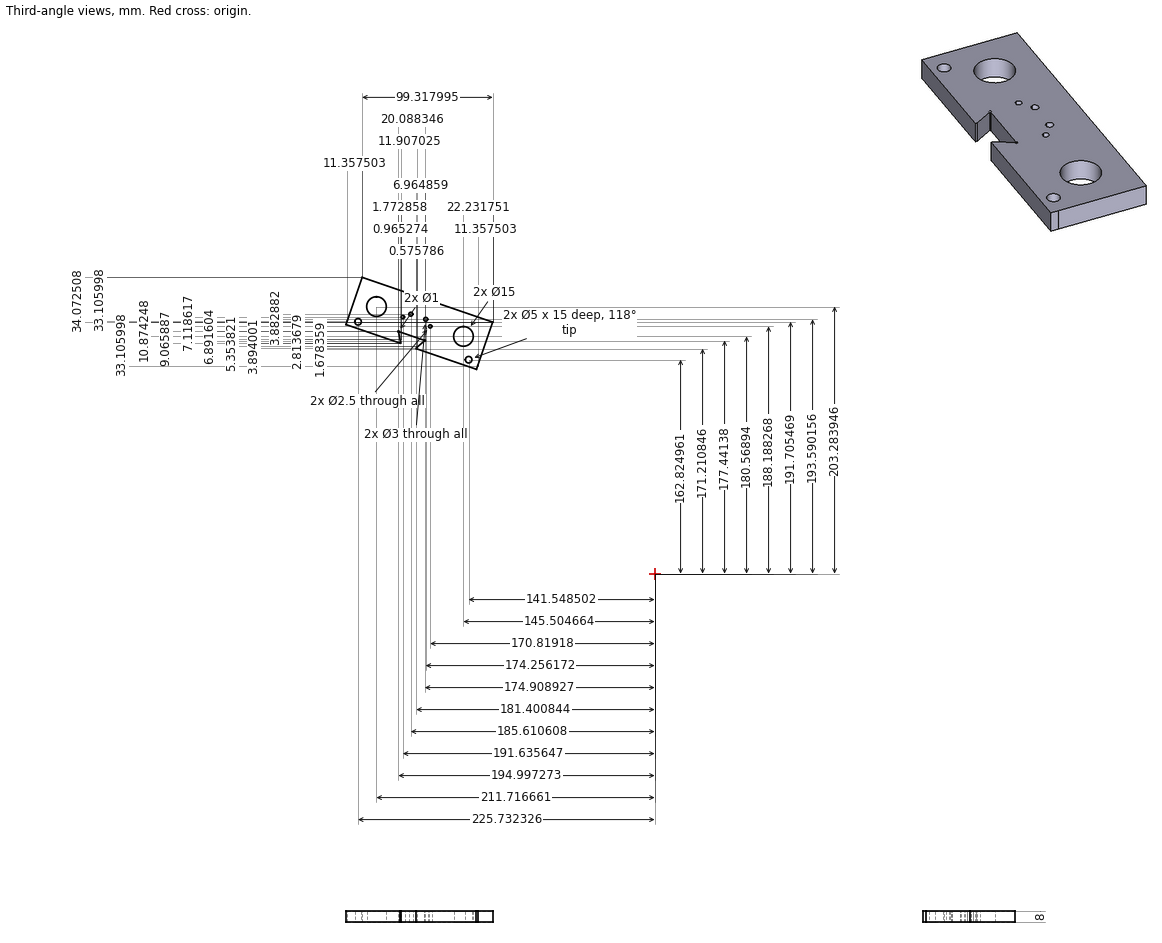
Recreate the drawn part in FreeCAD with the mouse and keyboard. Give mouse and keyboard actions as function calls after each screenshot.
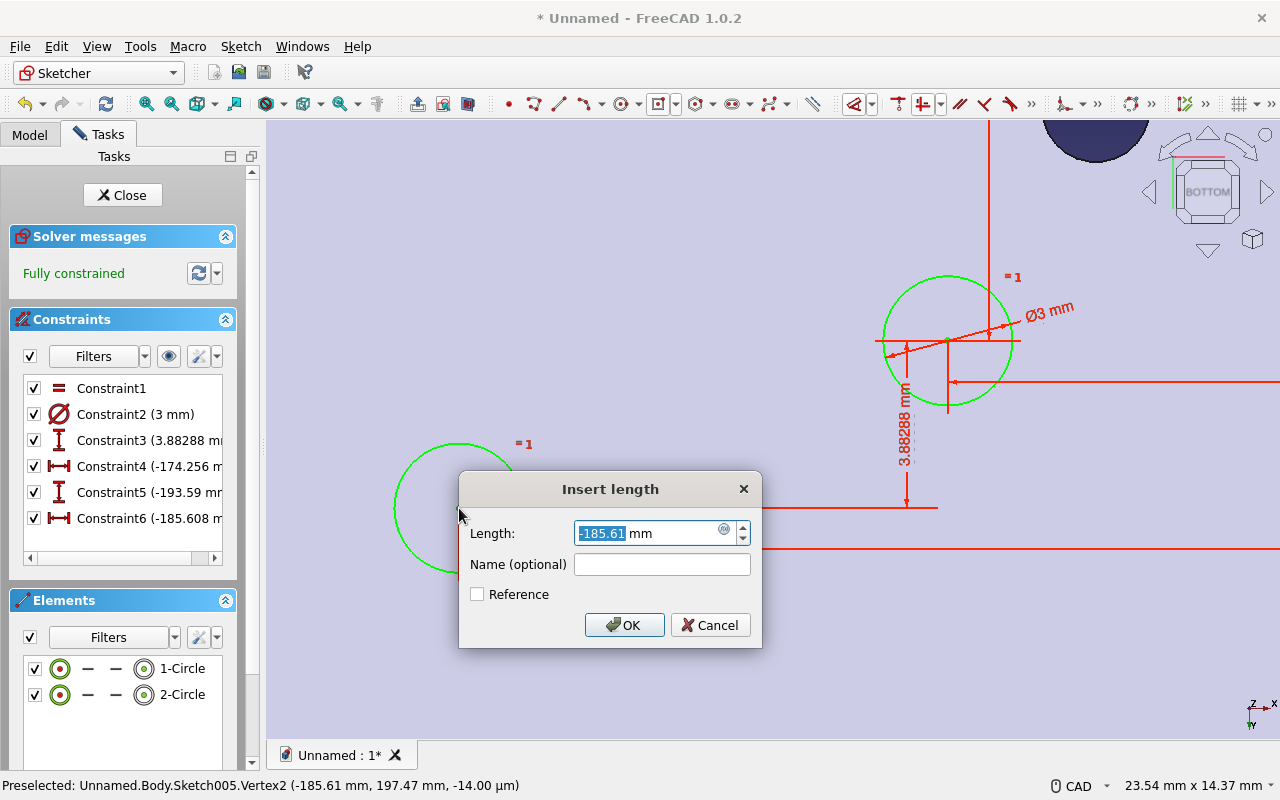
text(-185.610608)
key(Return)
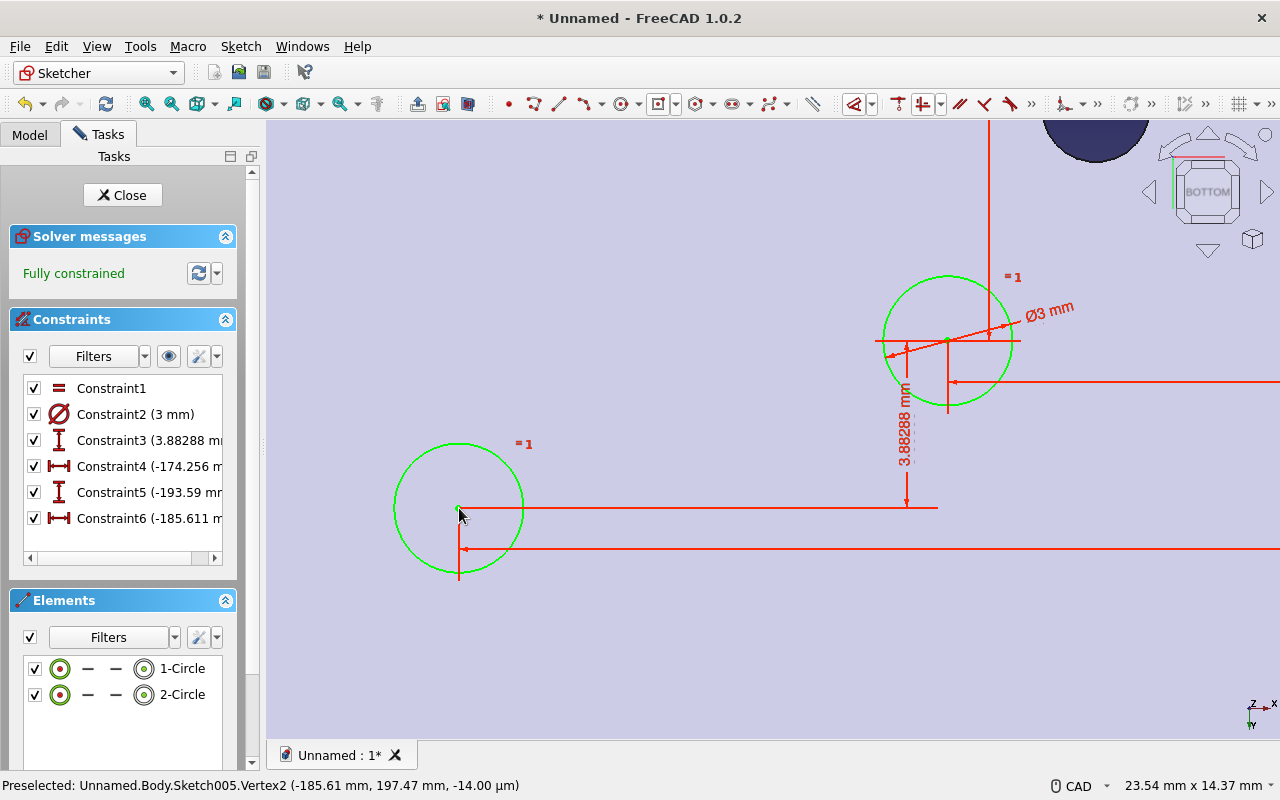
click(123, 195)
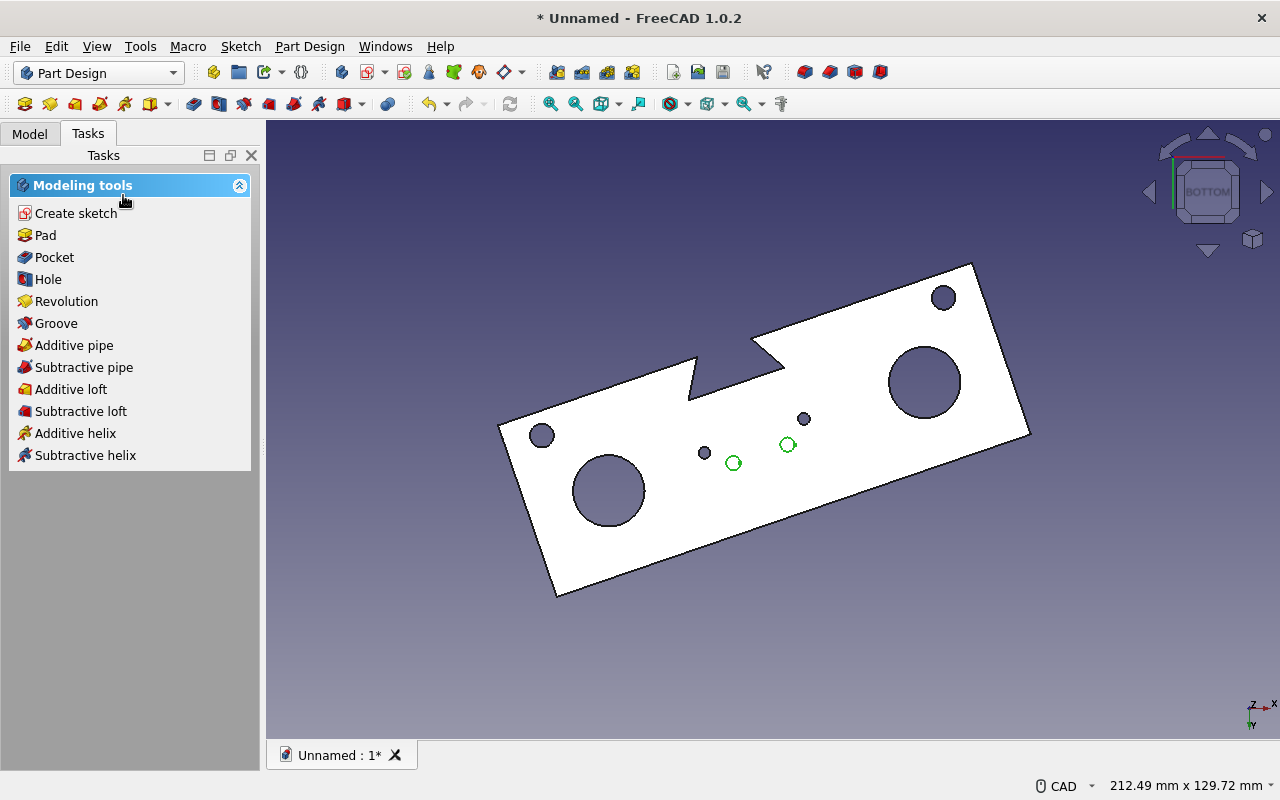
click(219, 104)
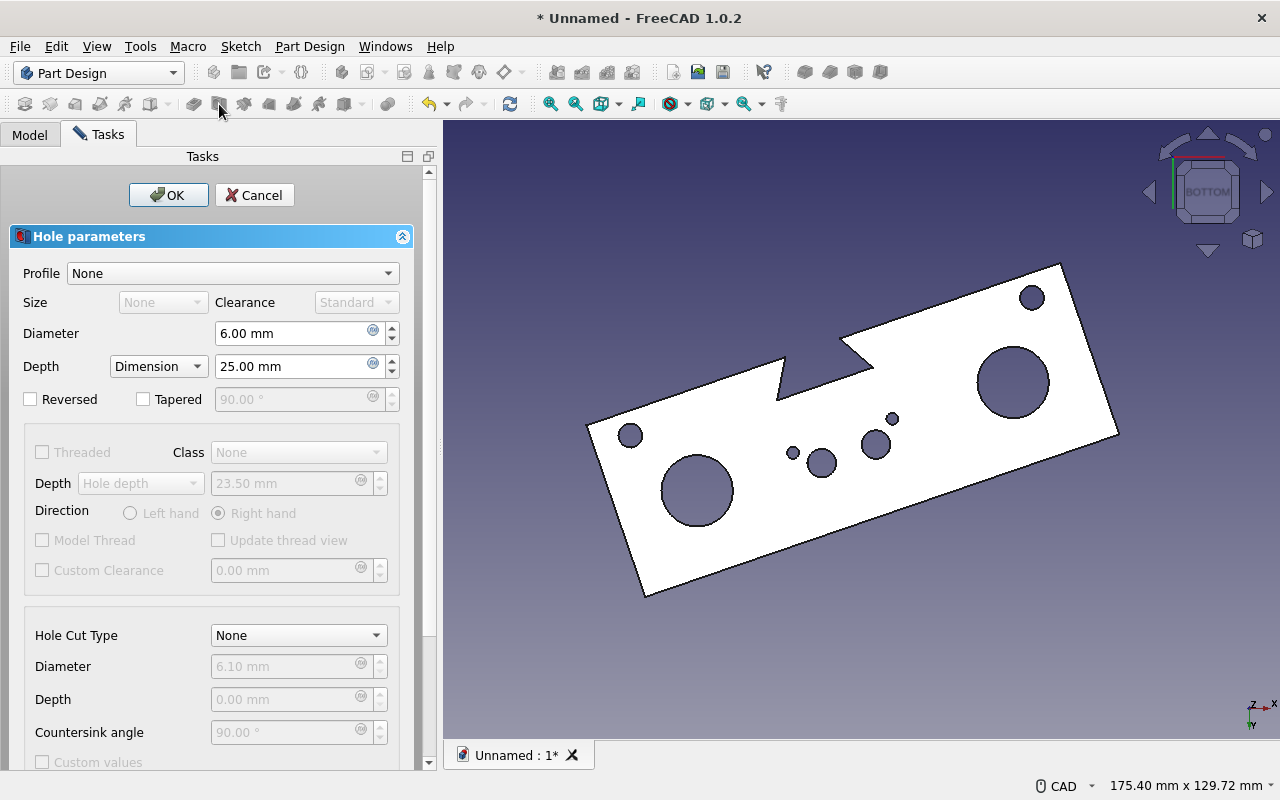
triple_click(300, 334)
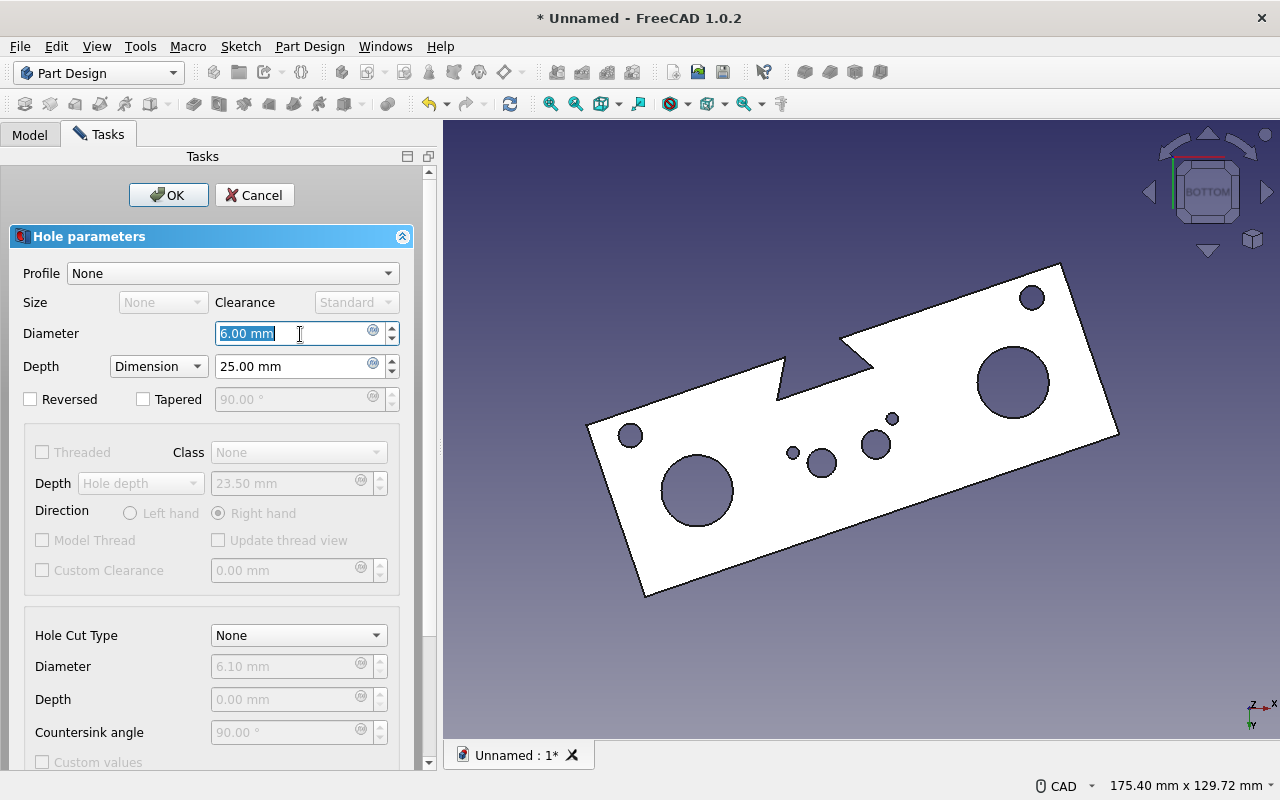
text(3)
key(Tab)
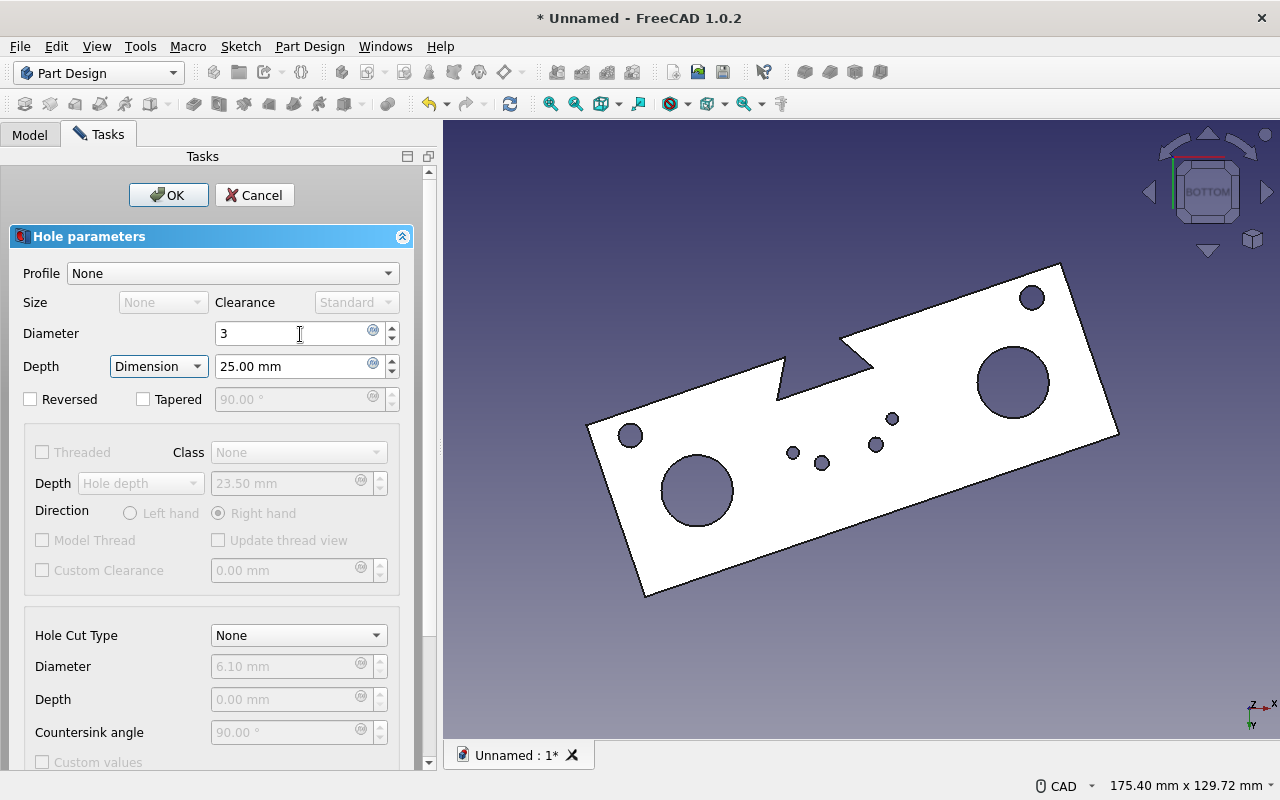
click(160, 366)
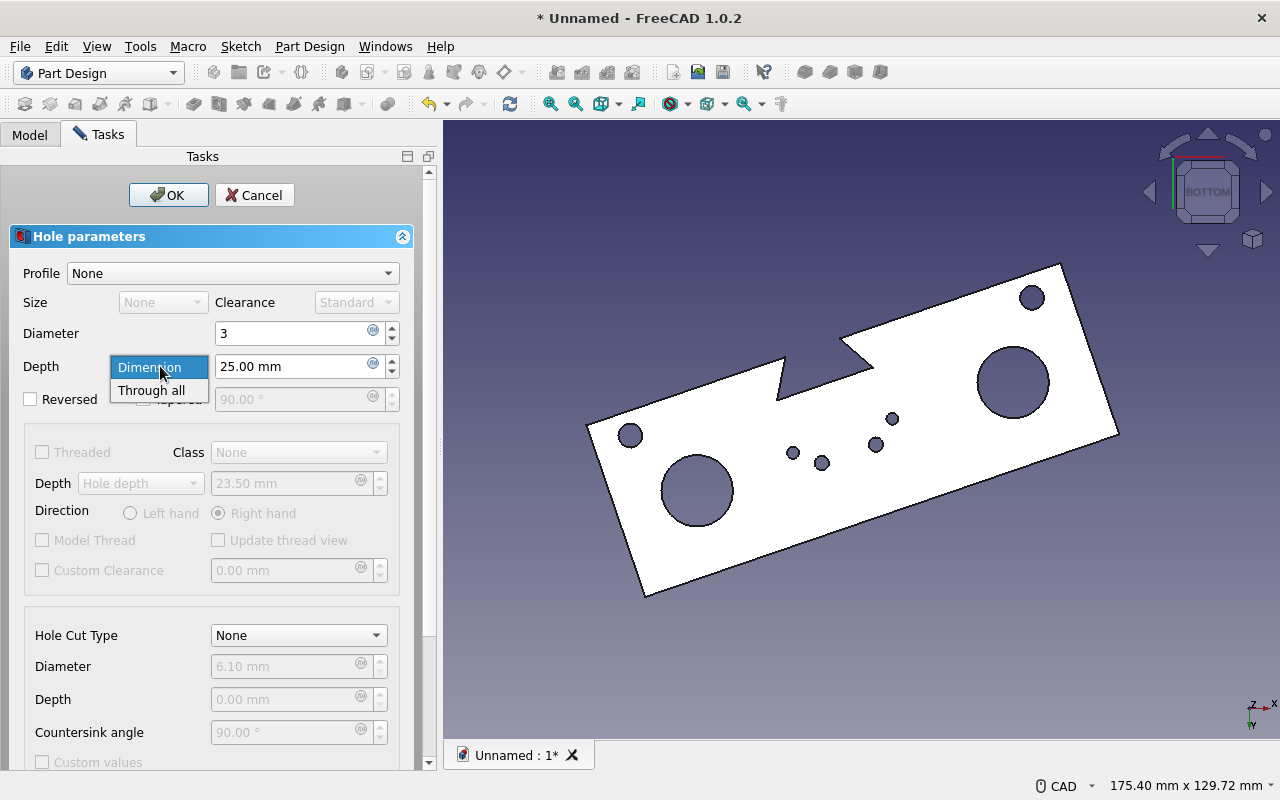
click(158, 390)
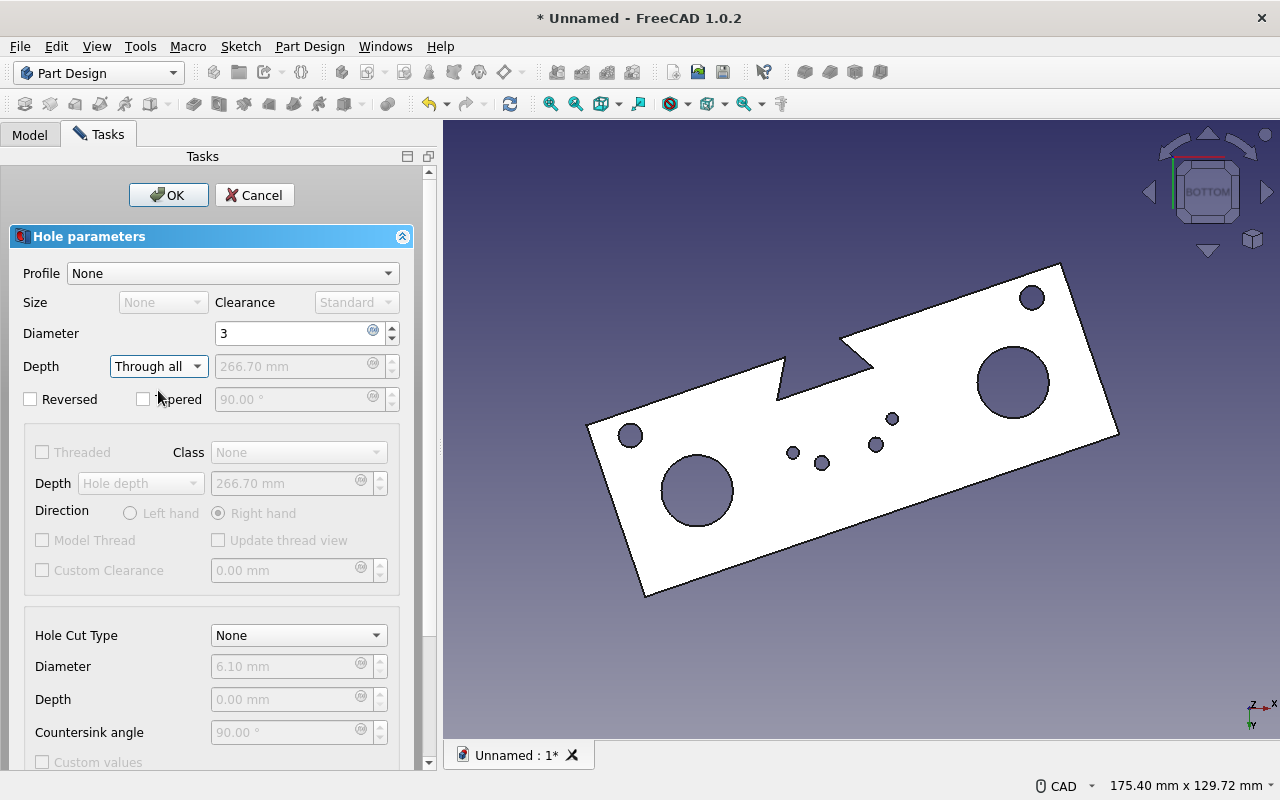
click(169, 195)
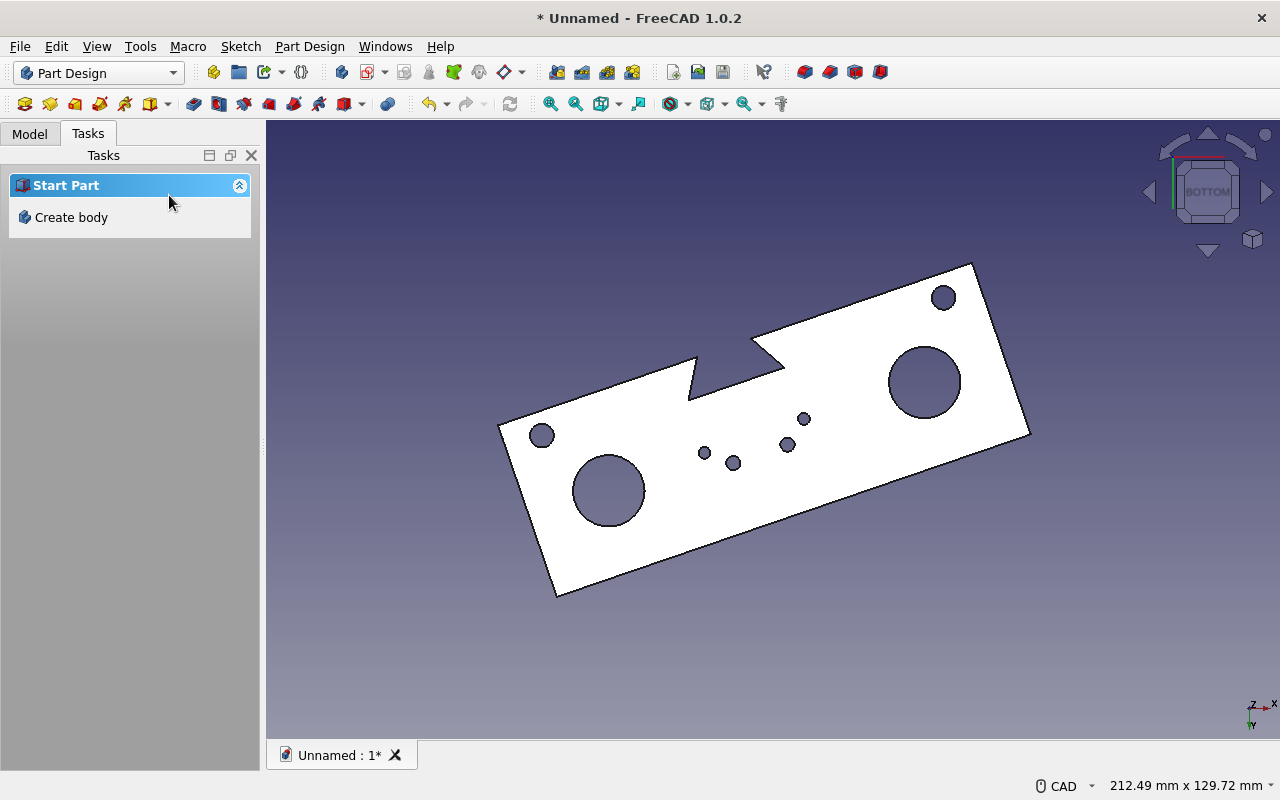
key(0)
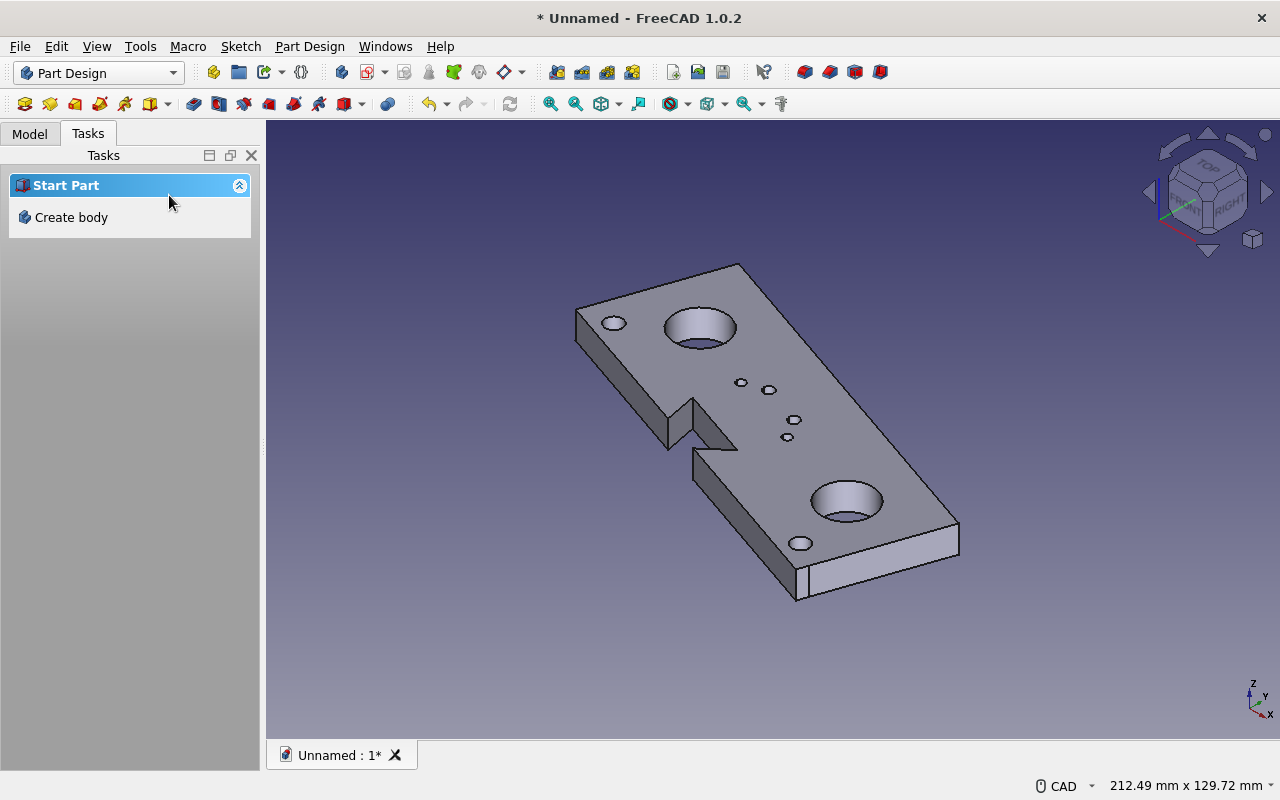
click(787, 466)